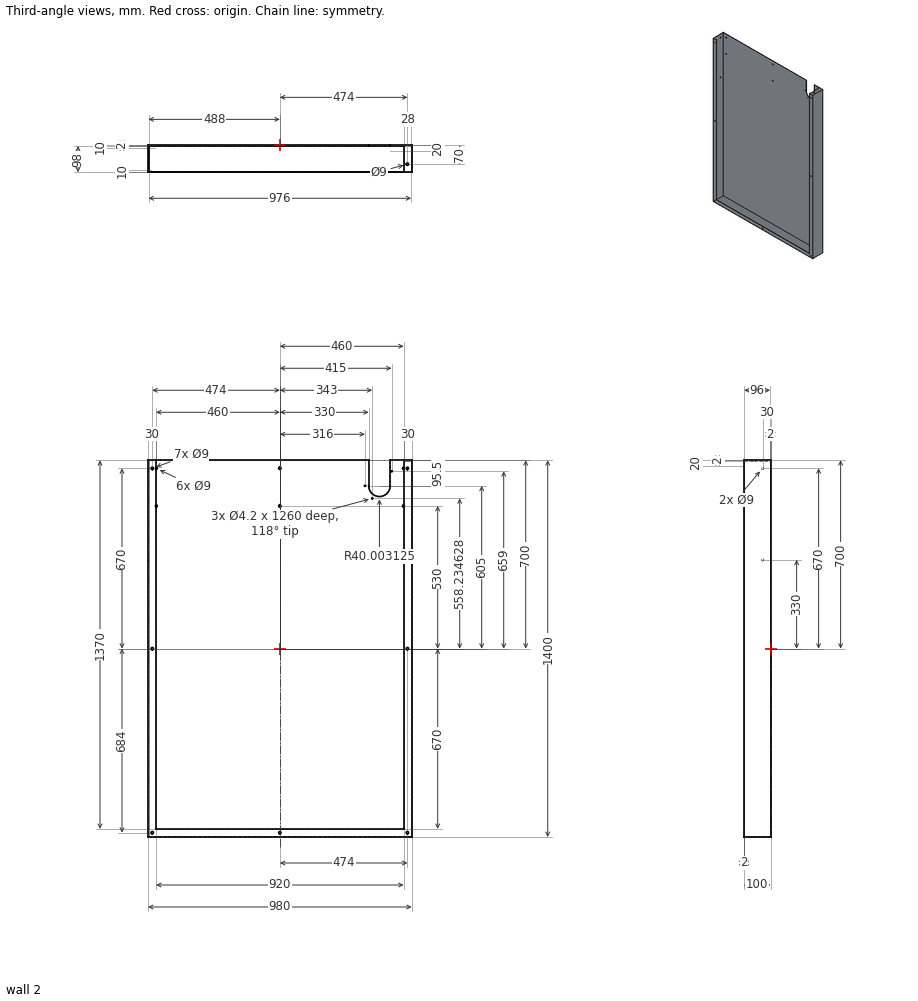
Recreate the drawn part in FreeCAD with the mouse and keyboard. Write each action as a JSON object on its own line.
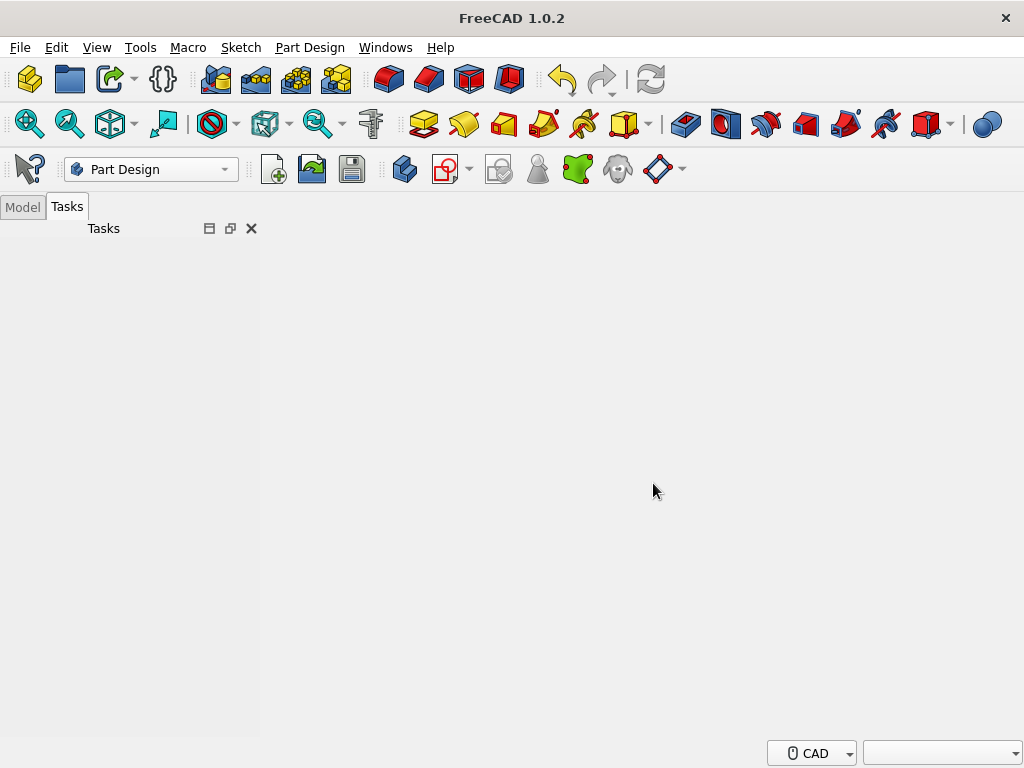
{"action": "left_click", "coordinate": [272, 170]}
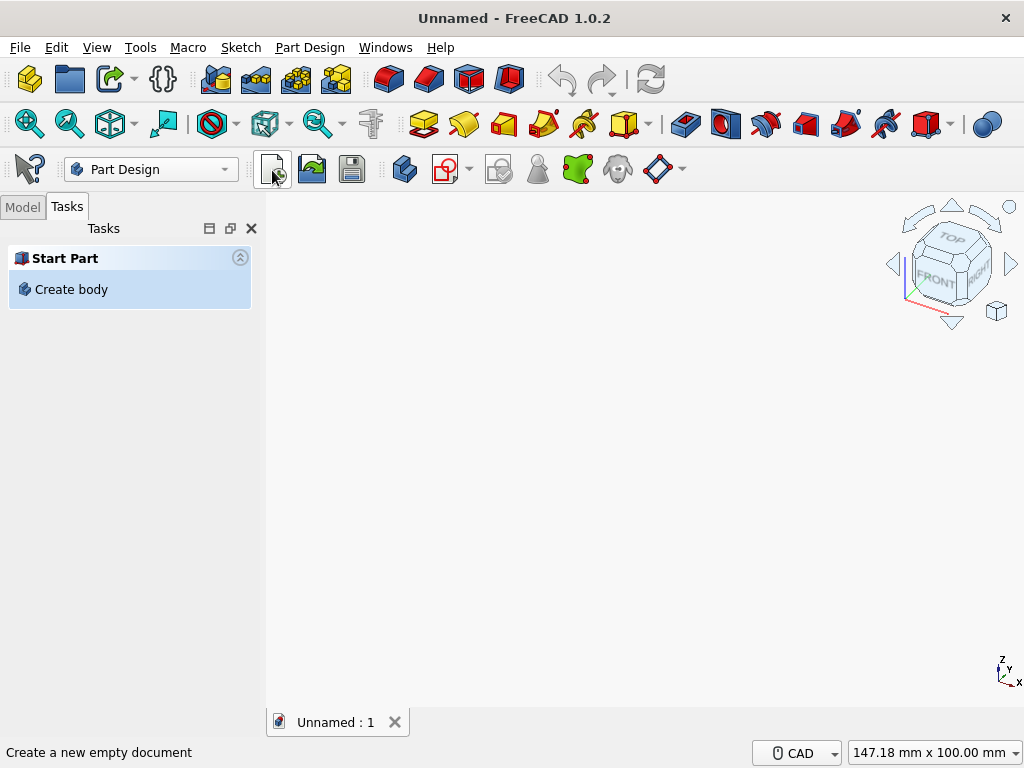
{"action": "left_click", "coordinate": [446, 170]}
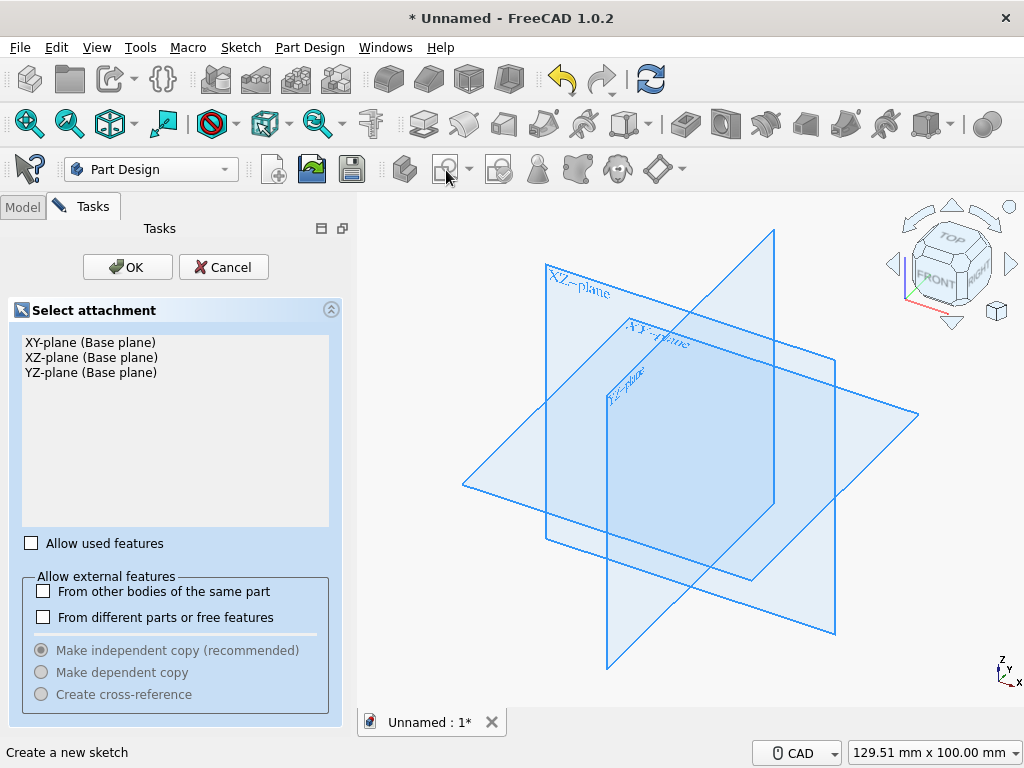
{"action": "left_click", "coordinate": [82, 358]}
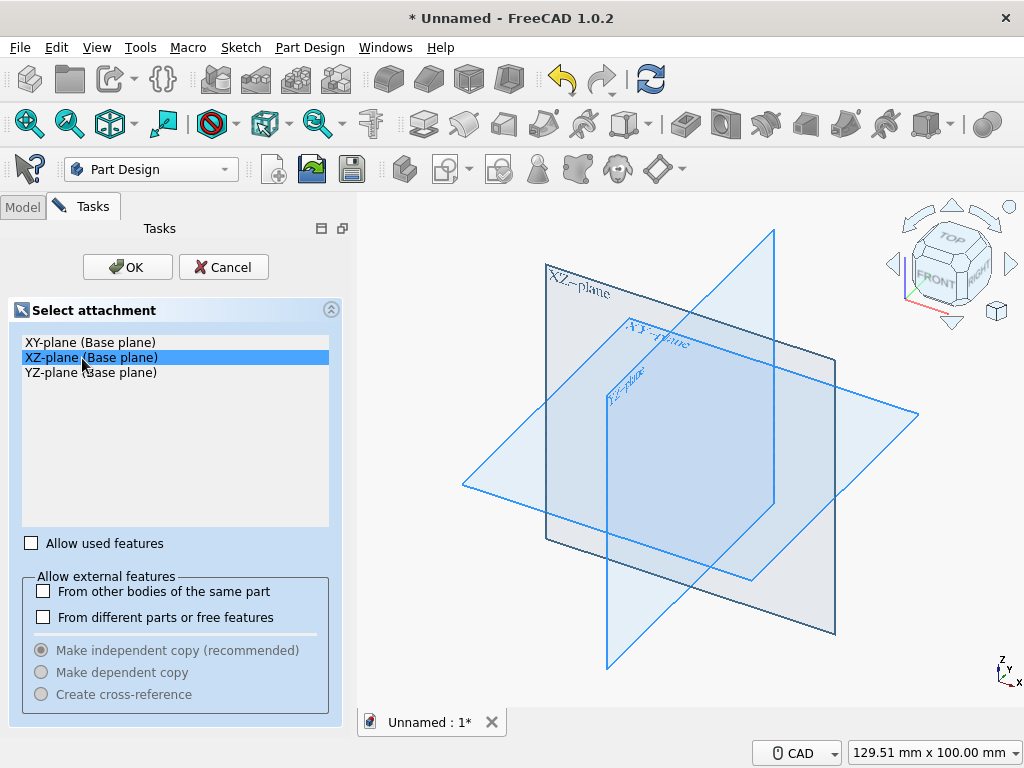
{"action": "left_click", "coordinate": [128, 267]}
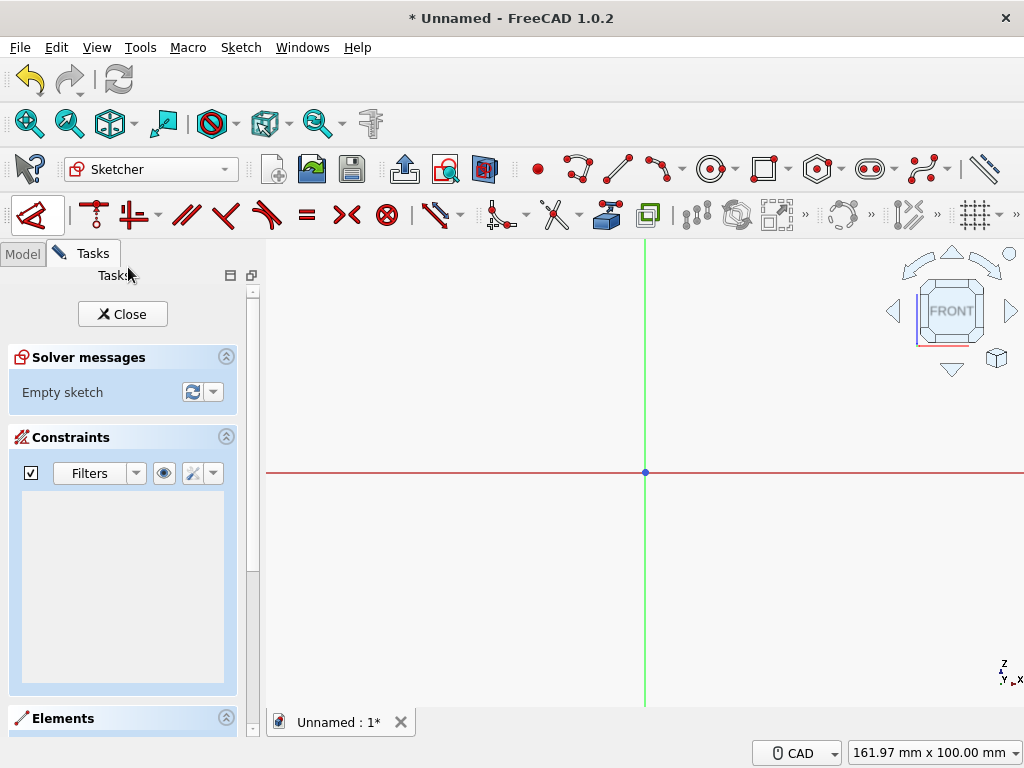
{"action": "scroll", "coordinate": [573, 473], "scroll_direction": "down", "scroll_amount": 15}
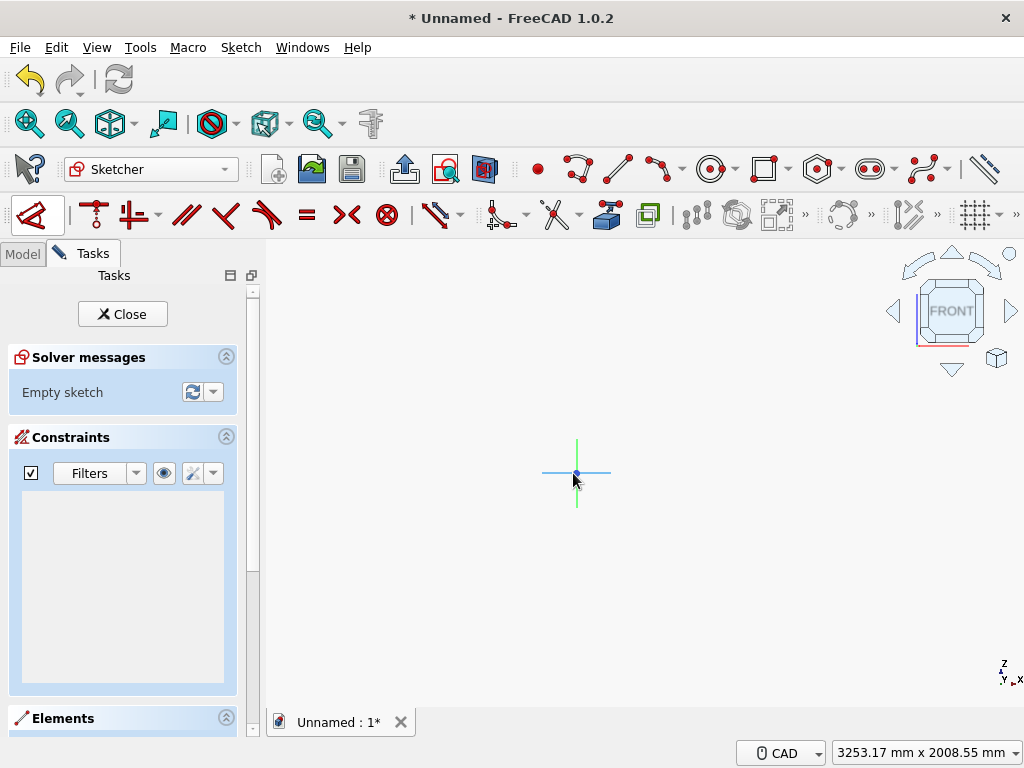
{"action": "left_click", "coordinate": [790, 170]}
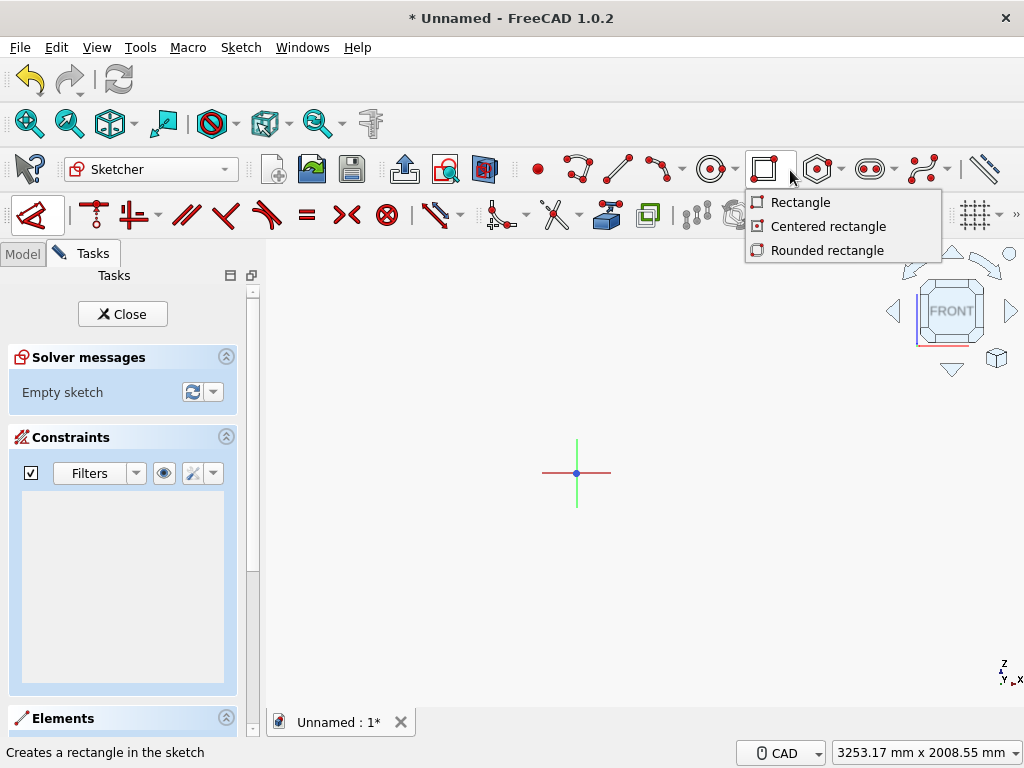
{"action": "left_click", "coordinate": [844, 226]}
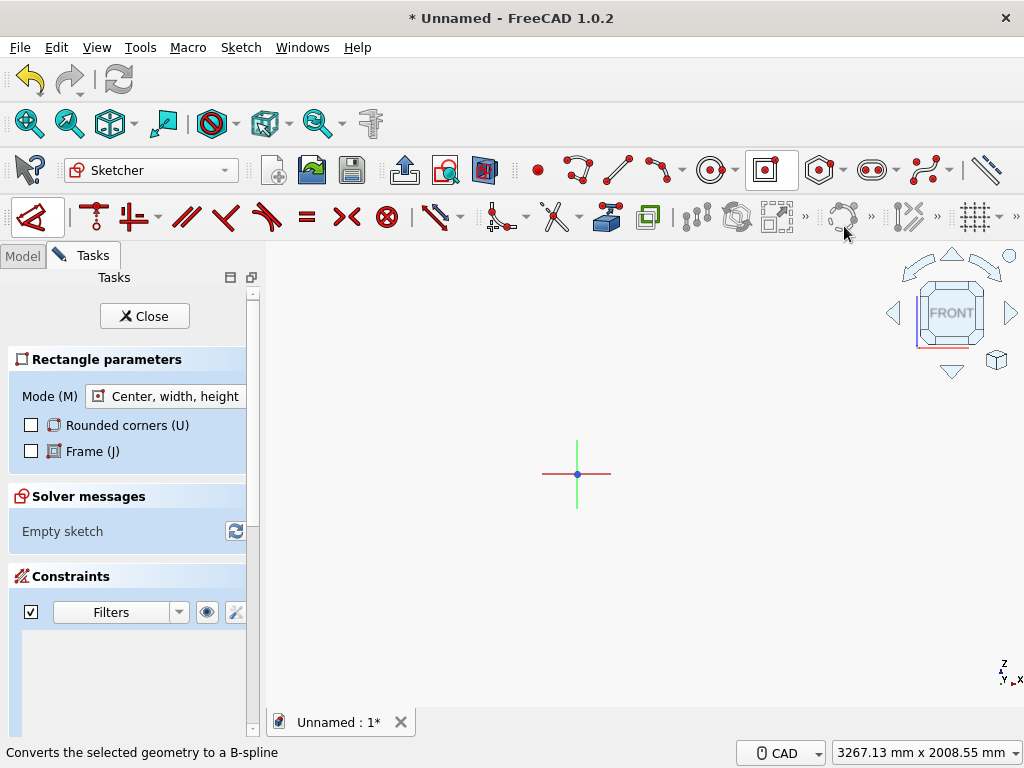
{"action": "left_click", "coordinate": [577, 474]}
{"action": "mouse_move", "coordinate": [691, 312]}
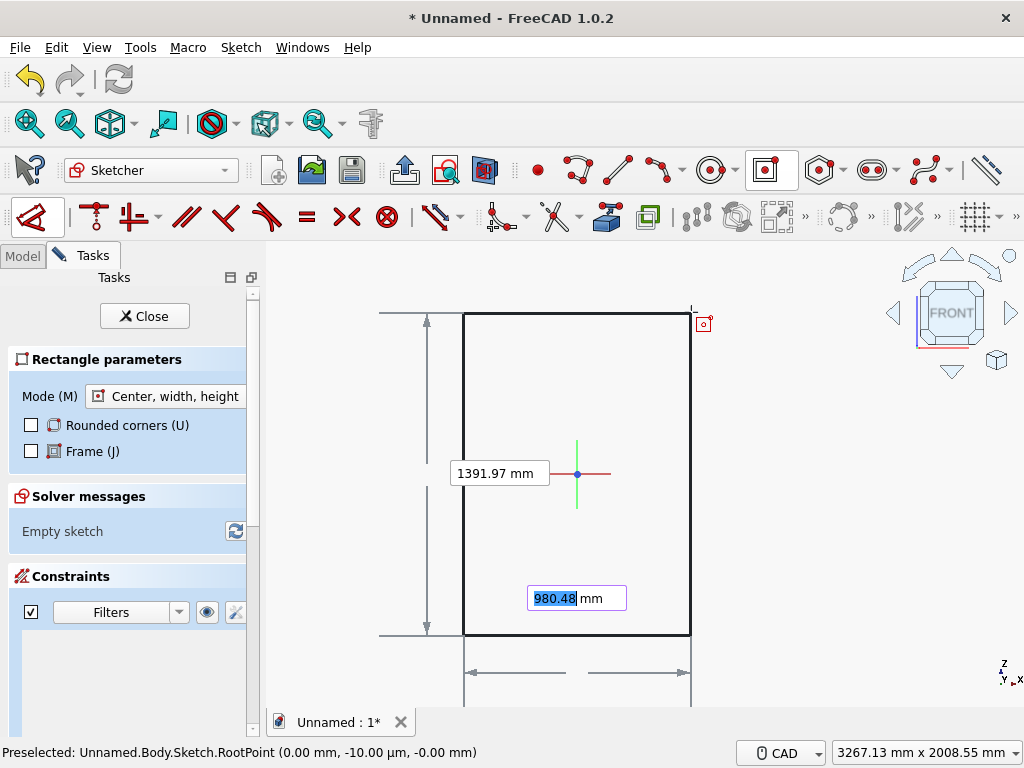
{"action": "type", "text": "980"}
{"action": "key", "text": "Tab"}
{"action": "type", "text": "1400"}
{"action": "key", "text": "Return"}
{"action": "key", "text": "Escape"}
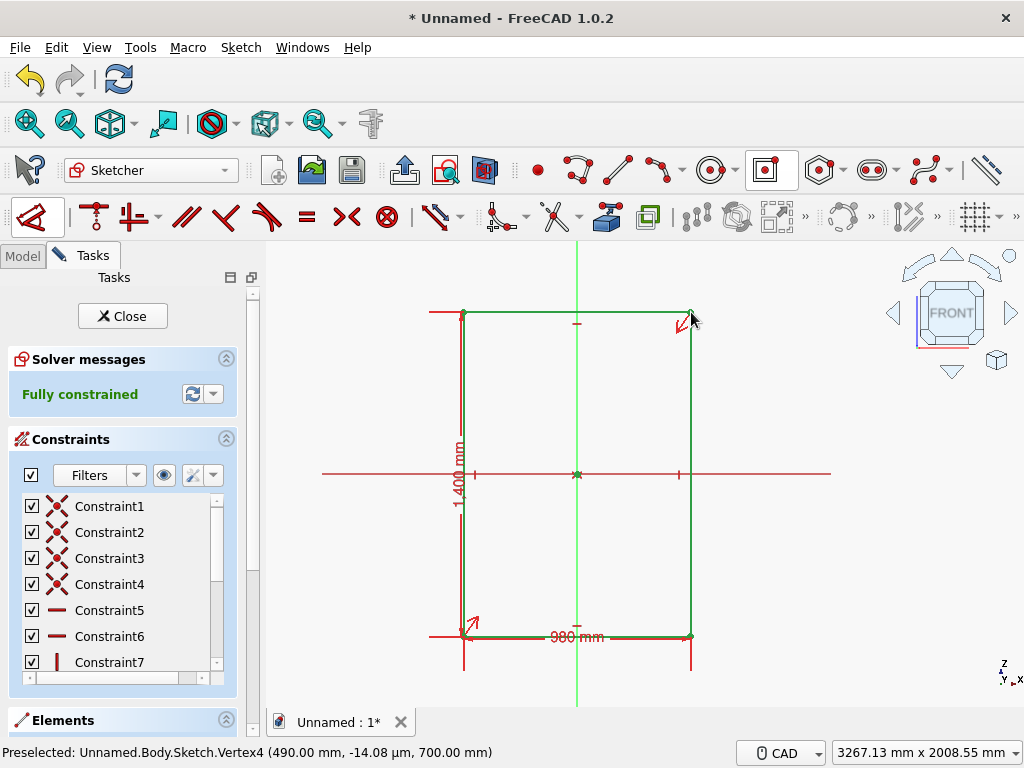
{"action": "left_click", "coordinate": [123, 316]}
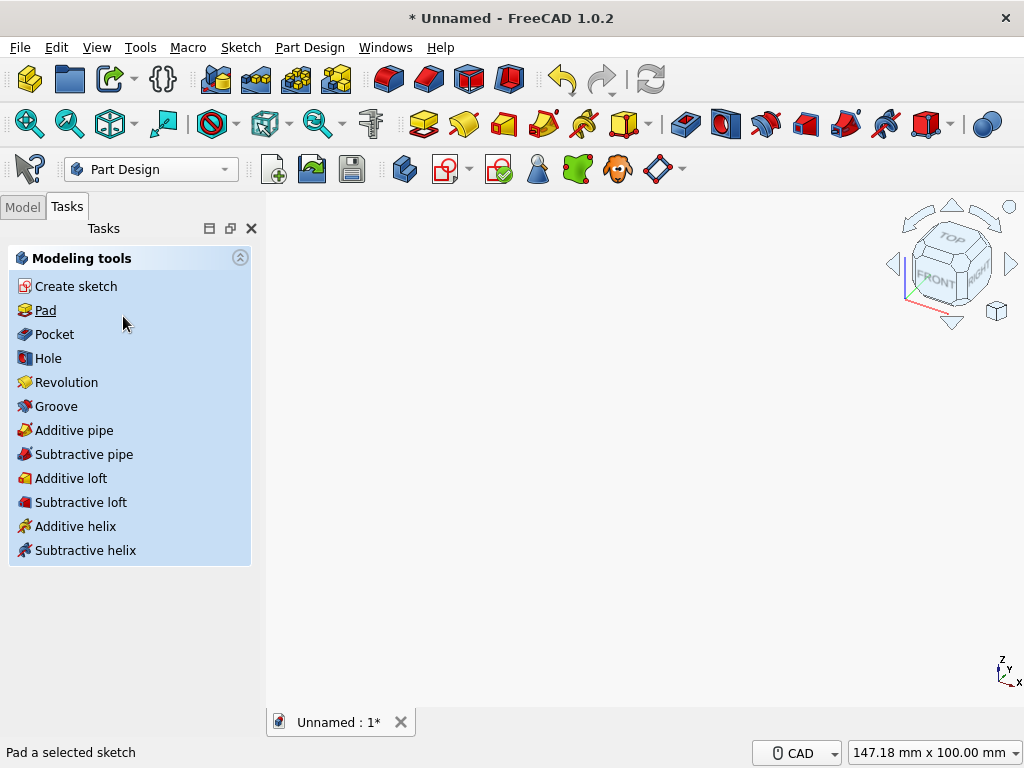
{"action": "left_click", "coordinate": [424, 124]}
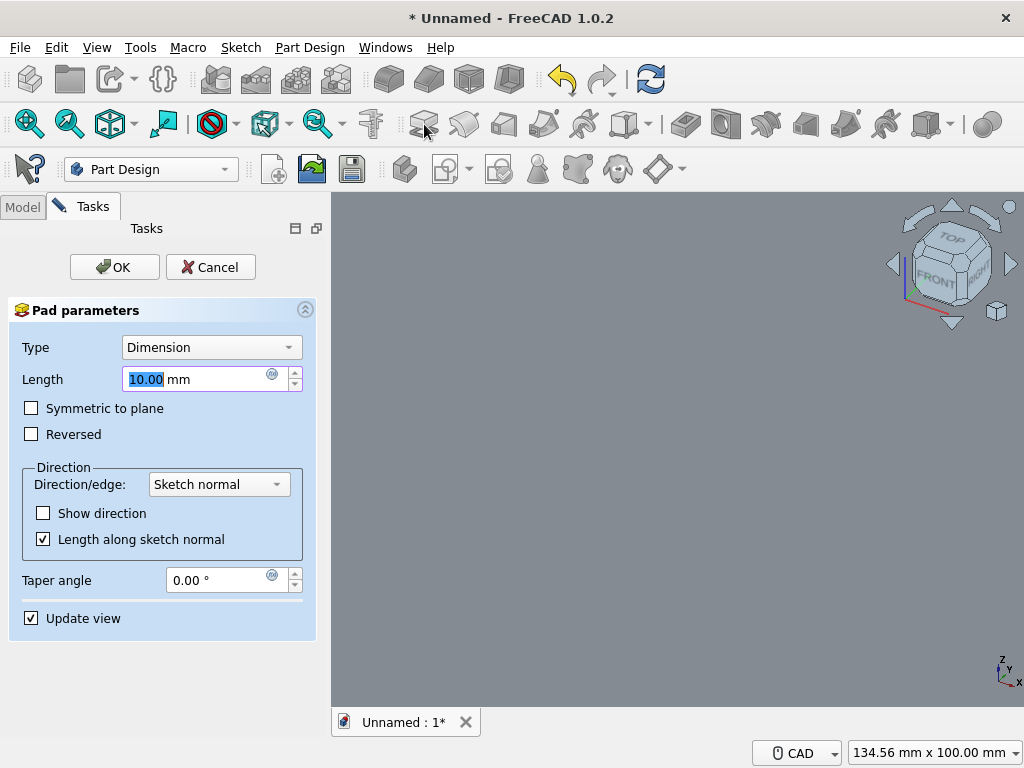
{"action": "type", "text": "100"}
{"action": "key", "text": "Tab"}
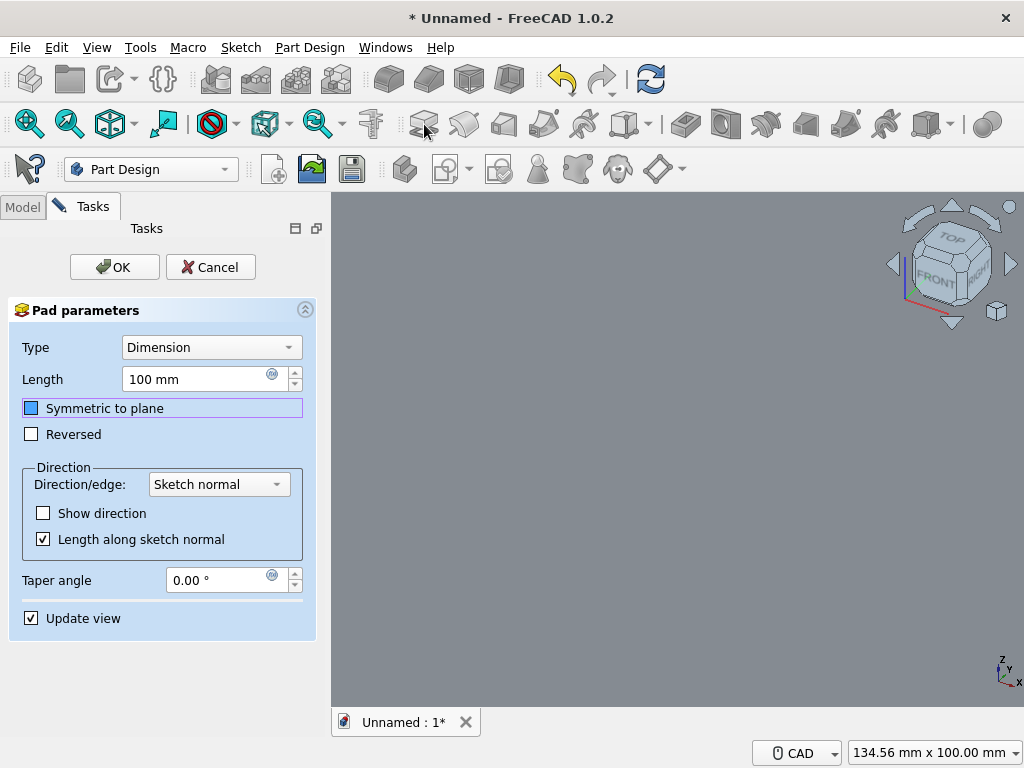
{"action": "left_click", "coordinate": [115, 267]}